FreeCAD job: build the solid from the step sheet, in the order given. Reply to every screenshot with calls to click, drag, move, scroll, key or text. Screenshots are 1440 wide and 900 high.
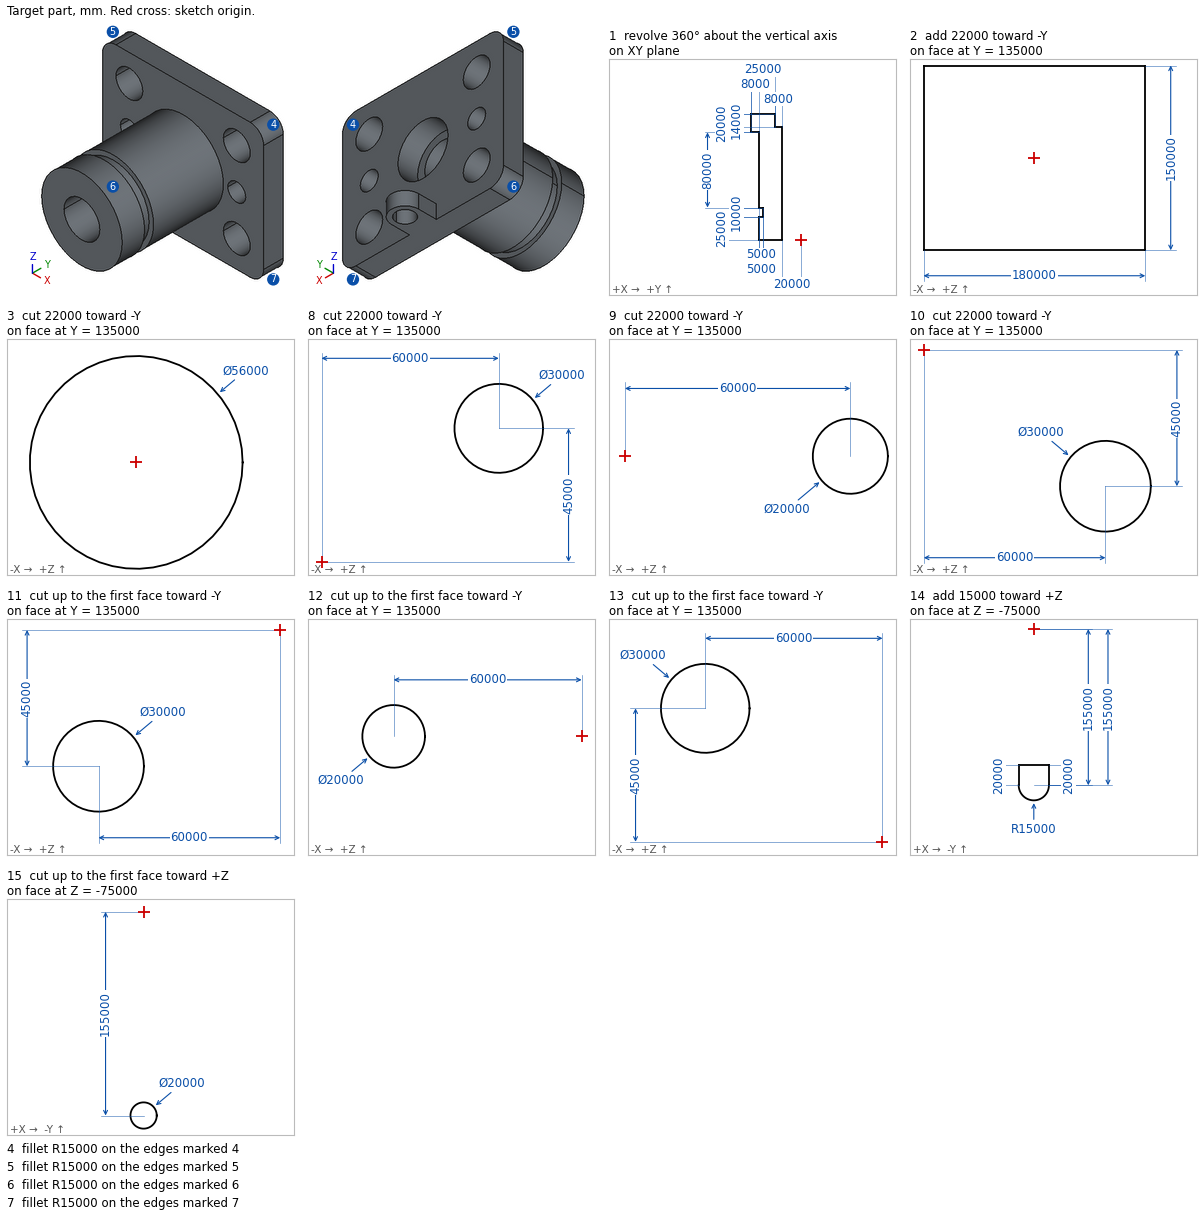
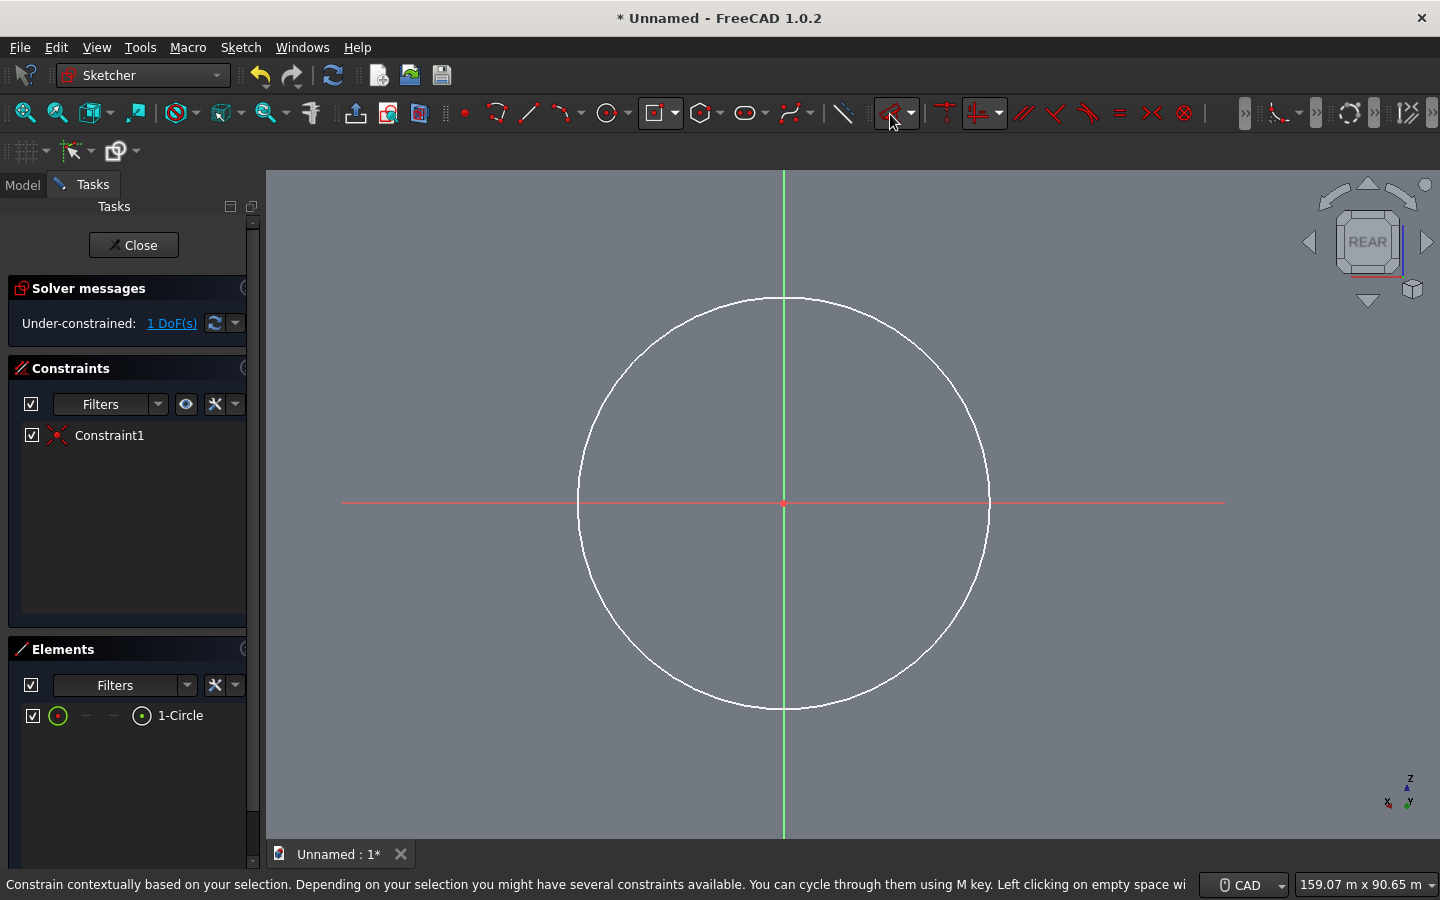
click(929, 357)
click(952, 334)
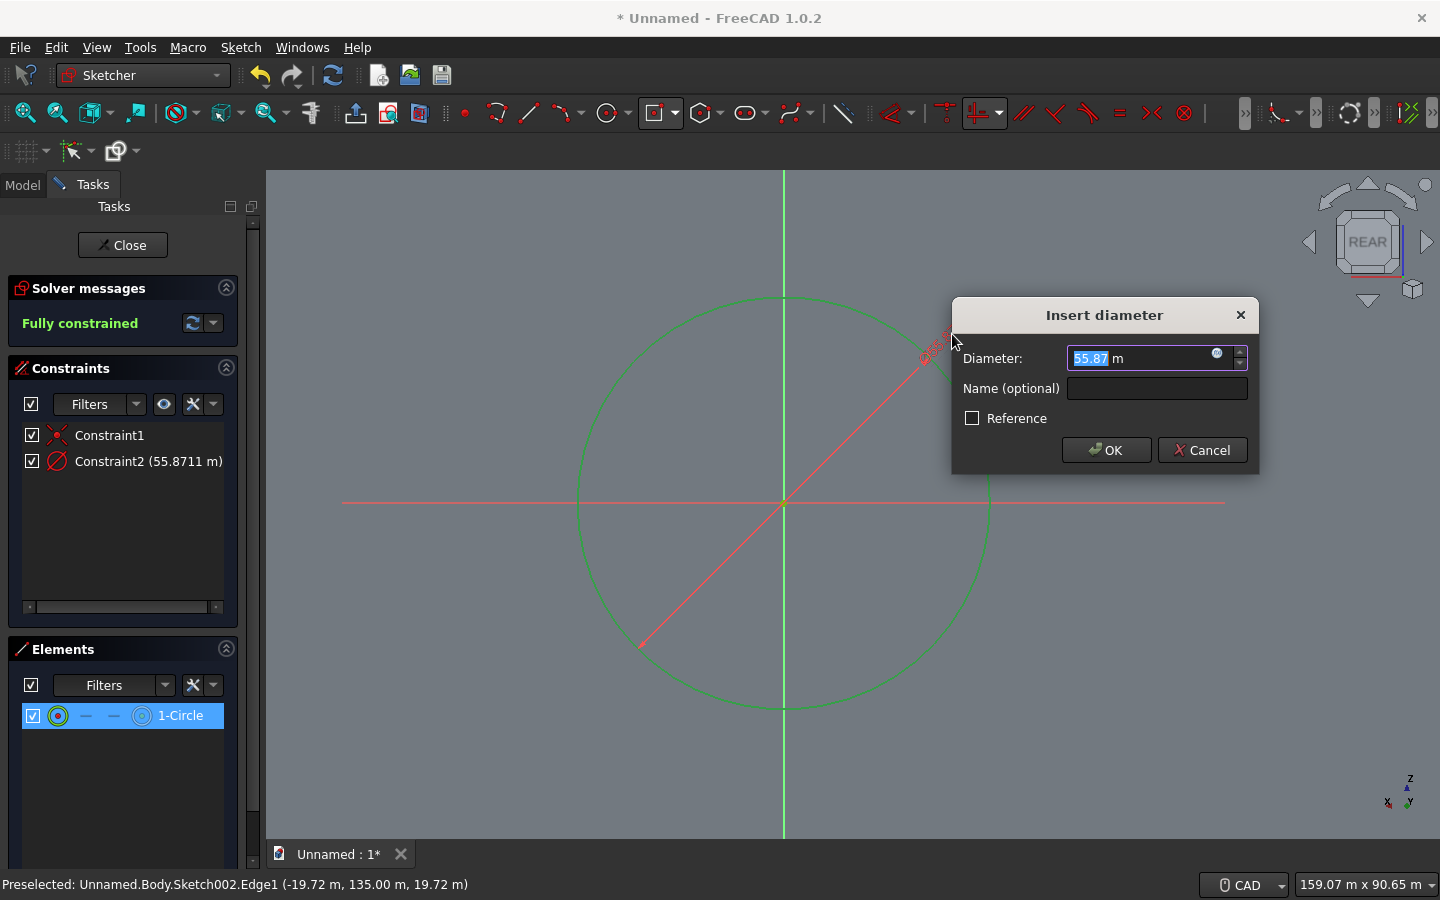
key(ctrl+a)
text(56000 mm)
key(Return)
key(Escape)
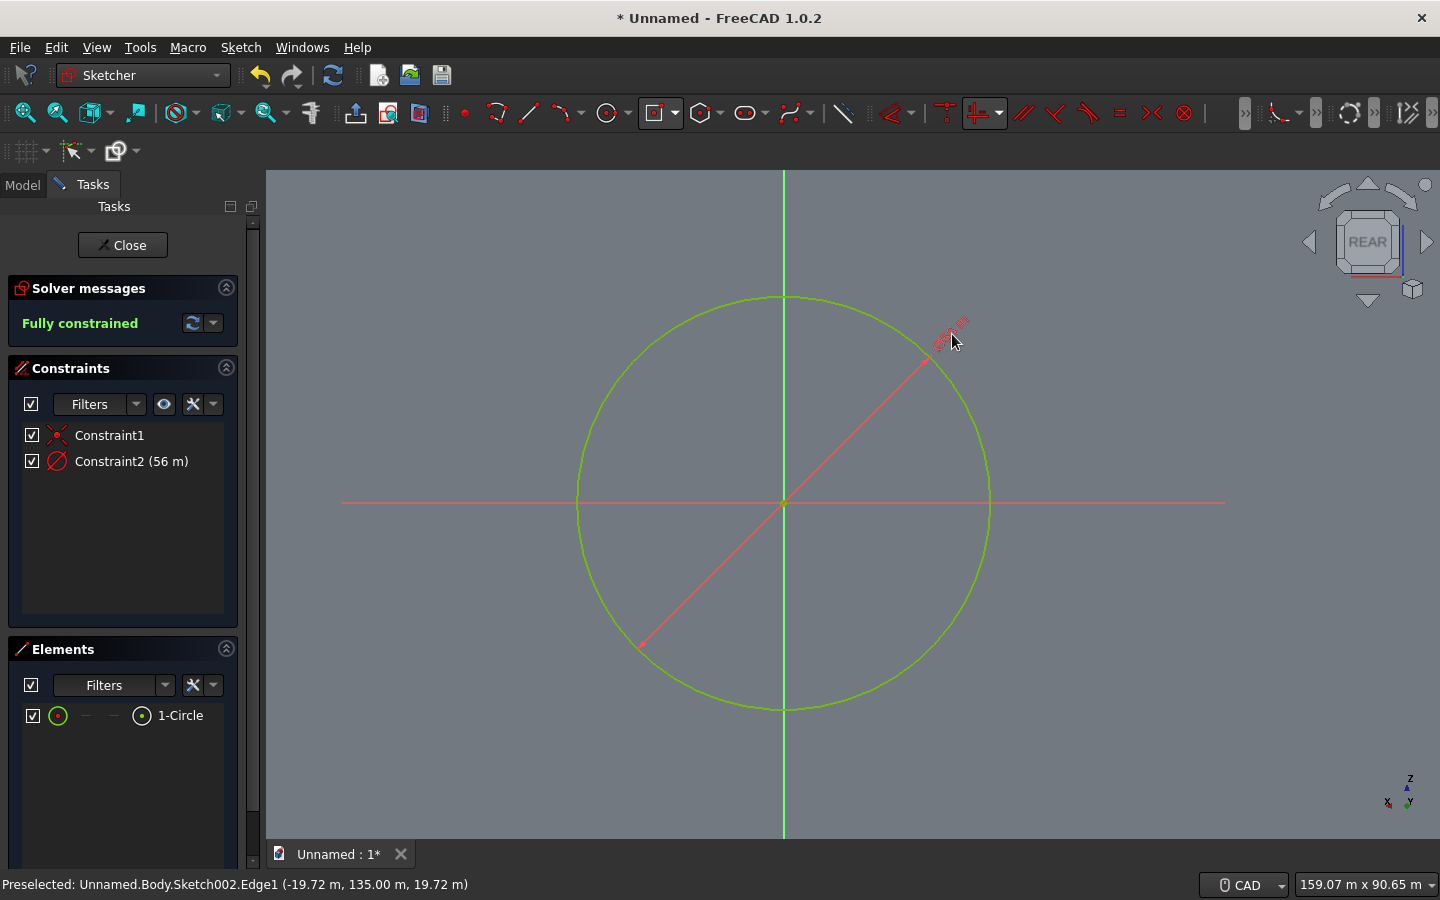
click(123, 245)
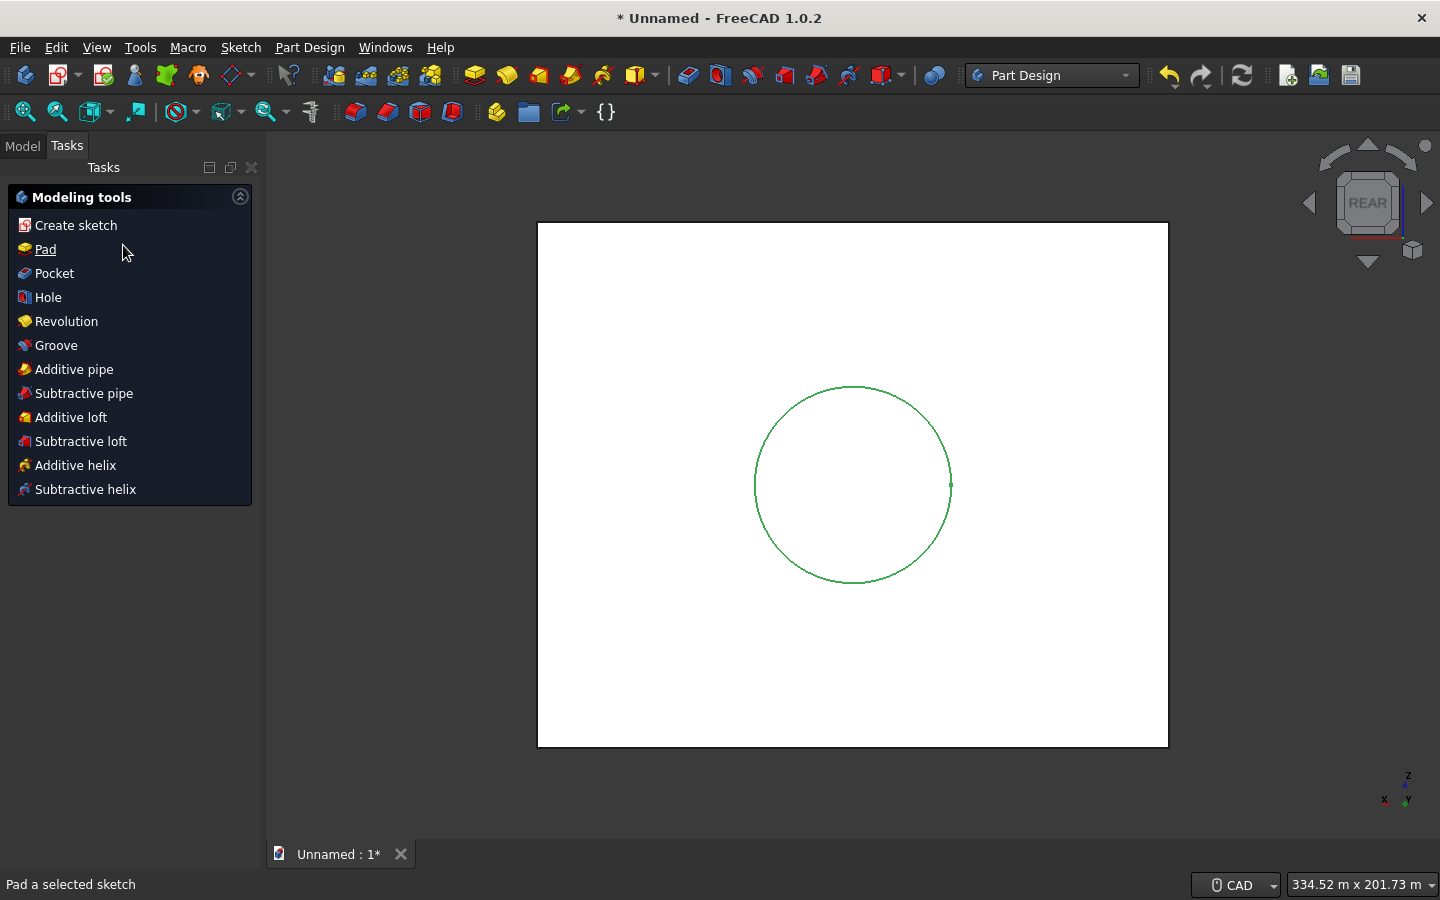
click(690, 76)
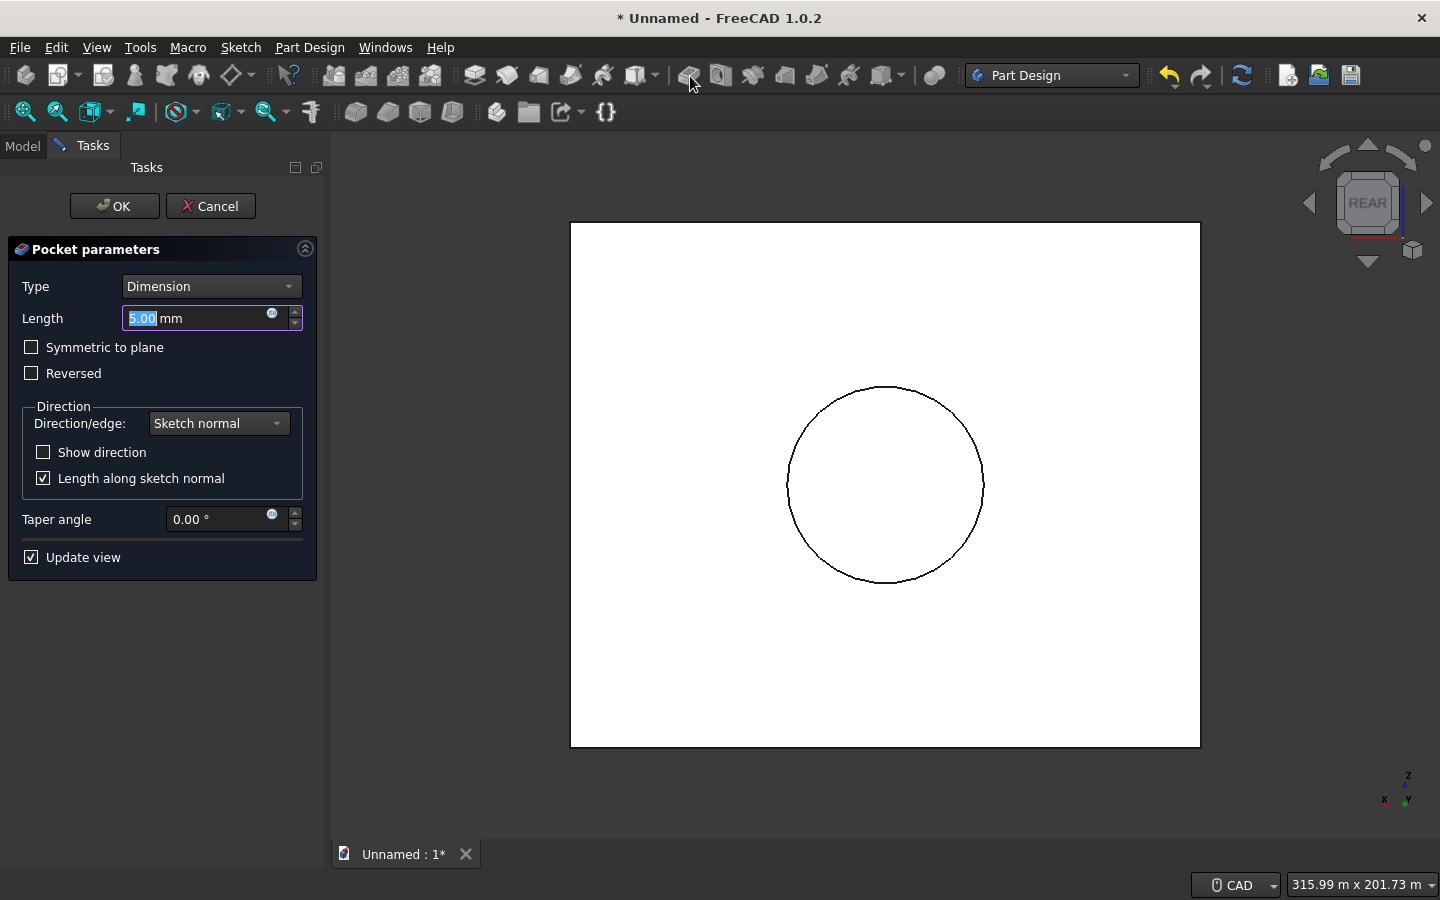
text(22000)
key(Tab)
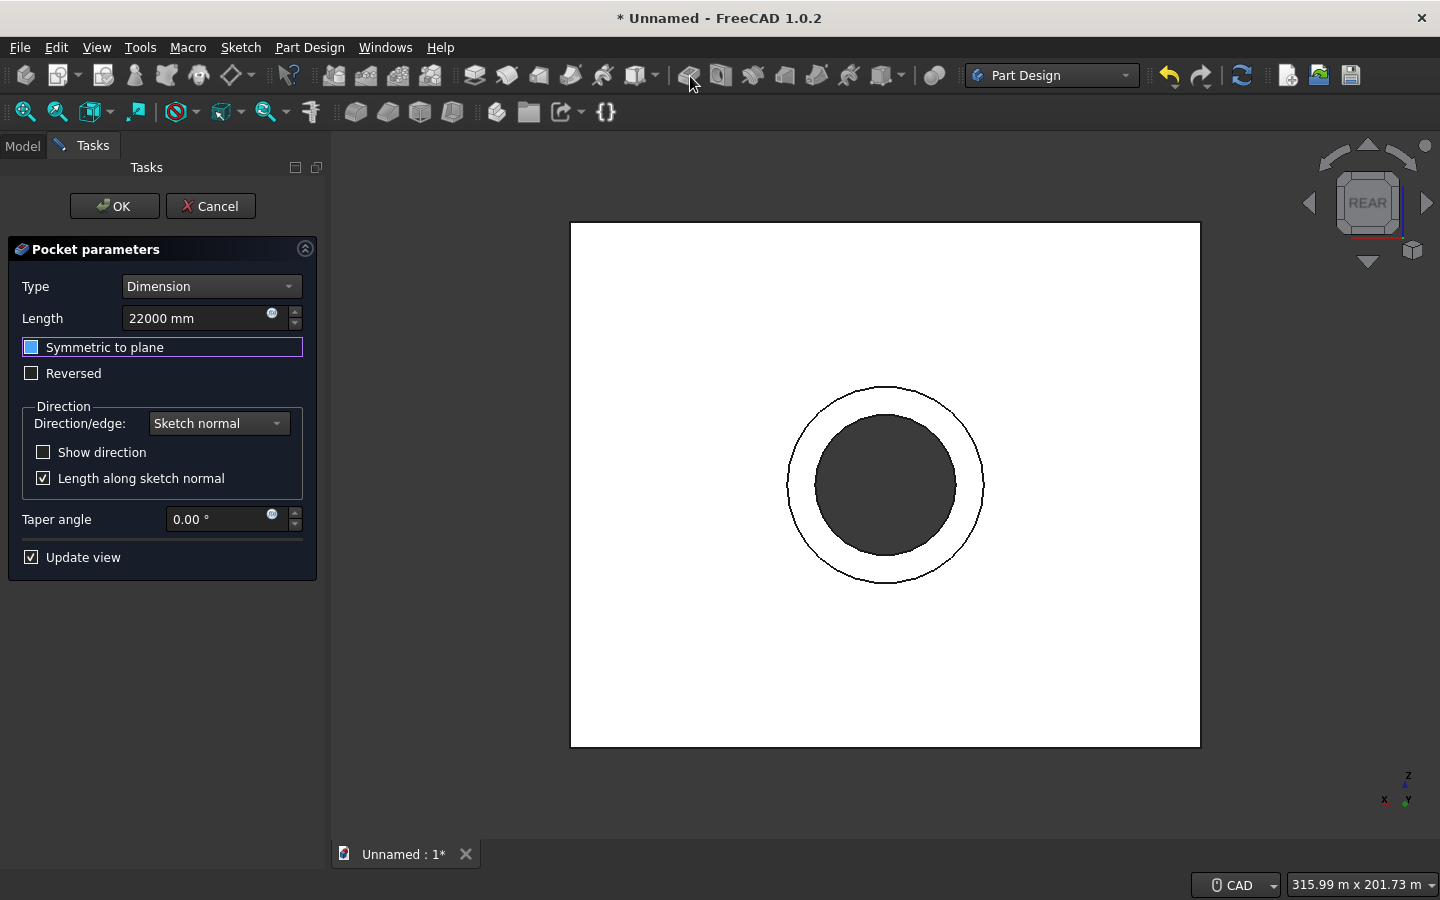
click(115, 206)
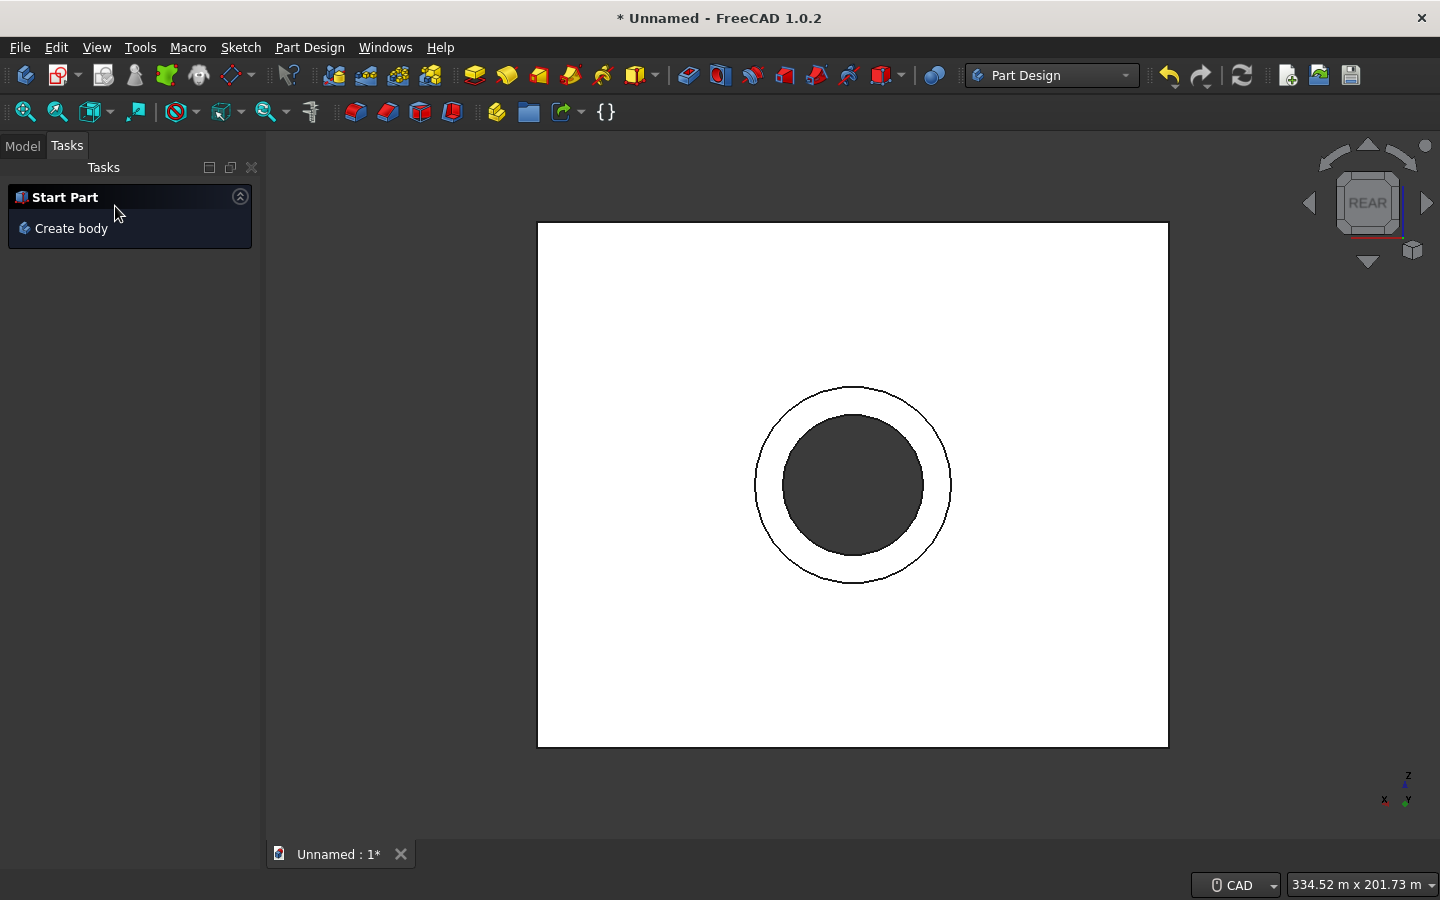
key(0)